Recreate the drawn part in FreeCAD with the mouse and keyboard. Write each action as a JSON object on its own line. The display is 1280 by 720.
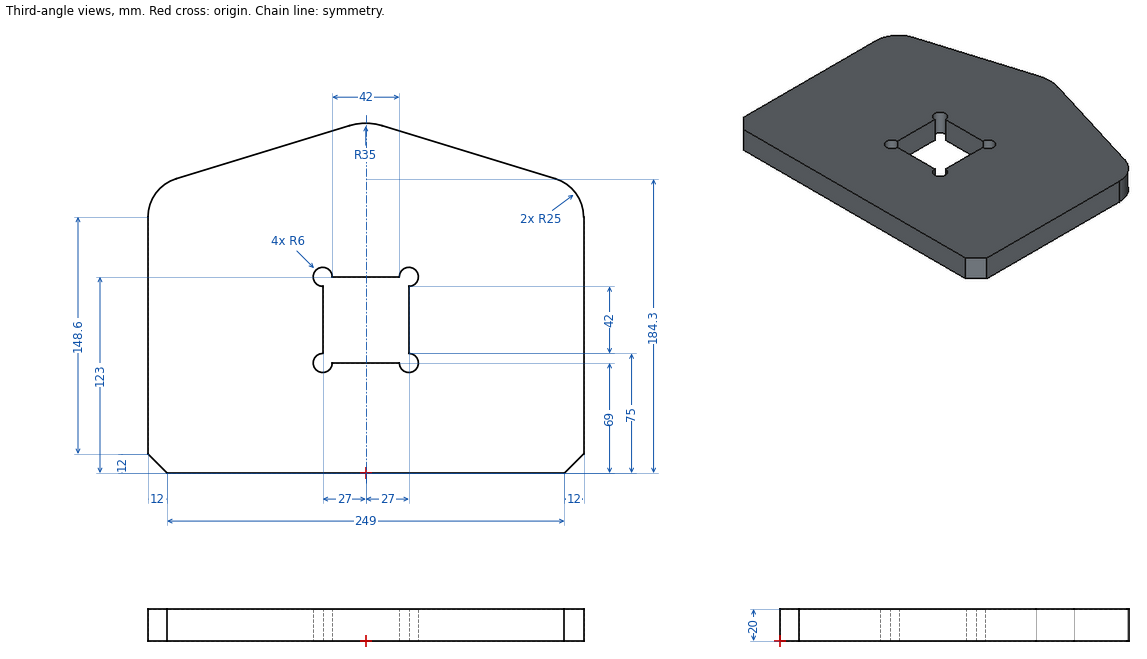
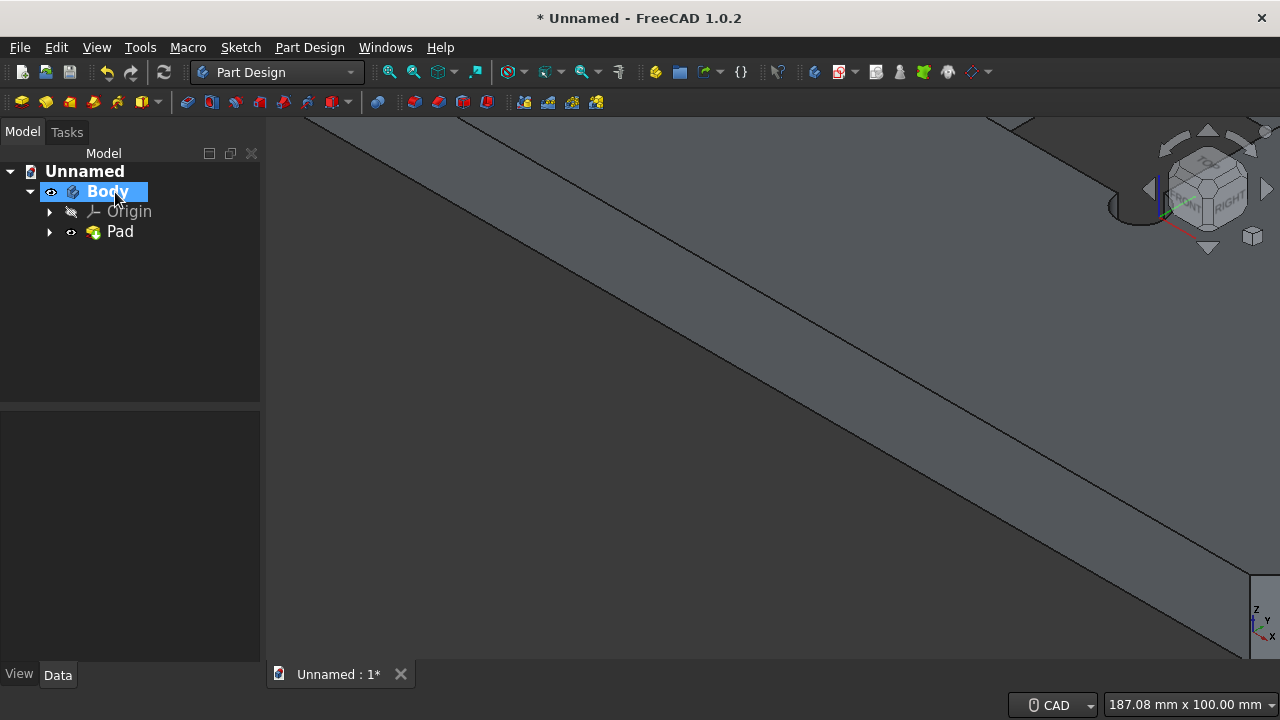
{"action": "left_click", "coordinate": [390, 72]}